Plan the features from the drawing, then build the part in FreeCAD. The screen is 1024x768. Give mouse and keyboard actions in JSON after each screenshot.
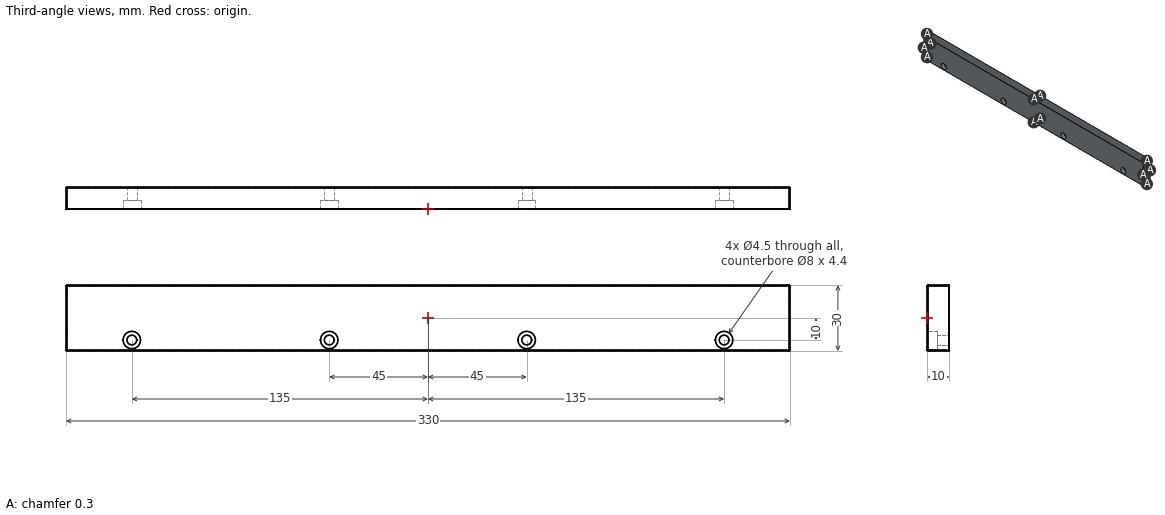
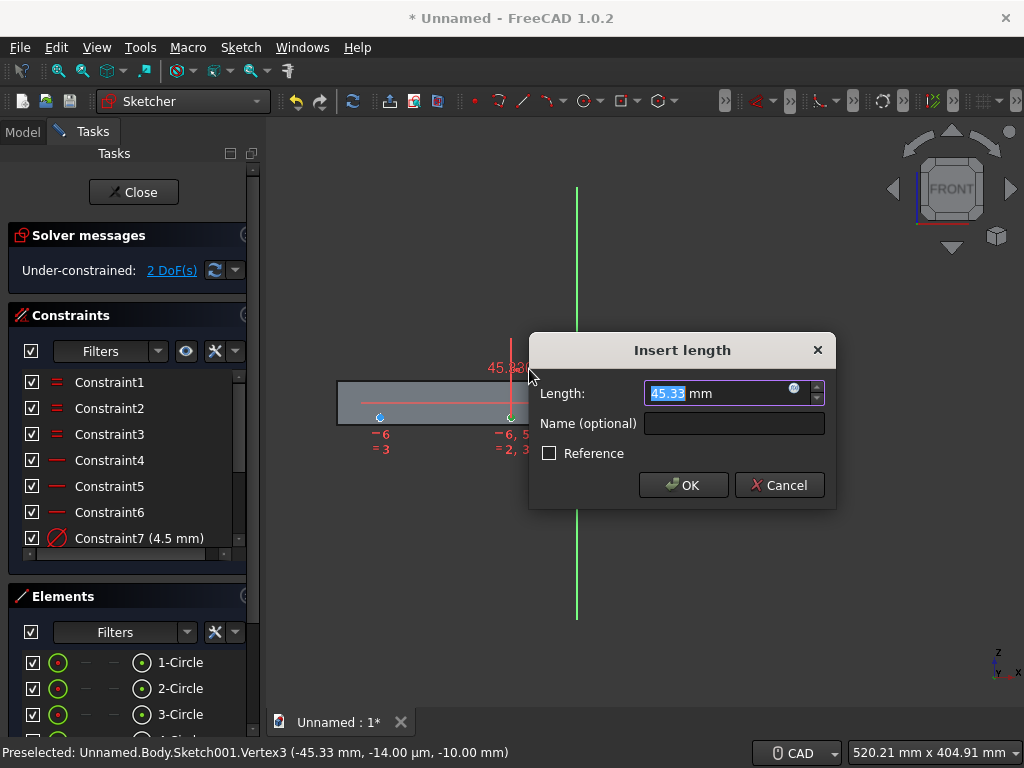
{"action": "type", "text": "45"}
{"action": "key", "text": "Return"}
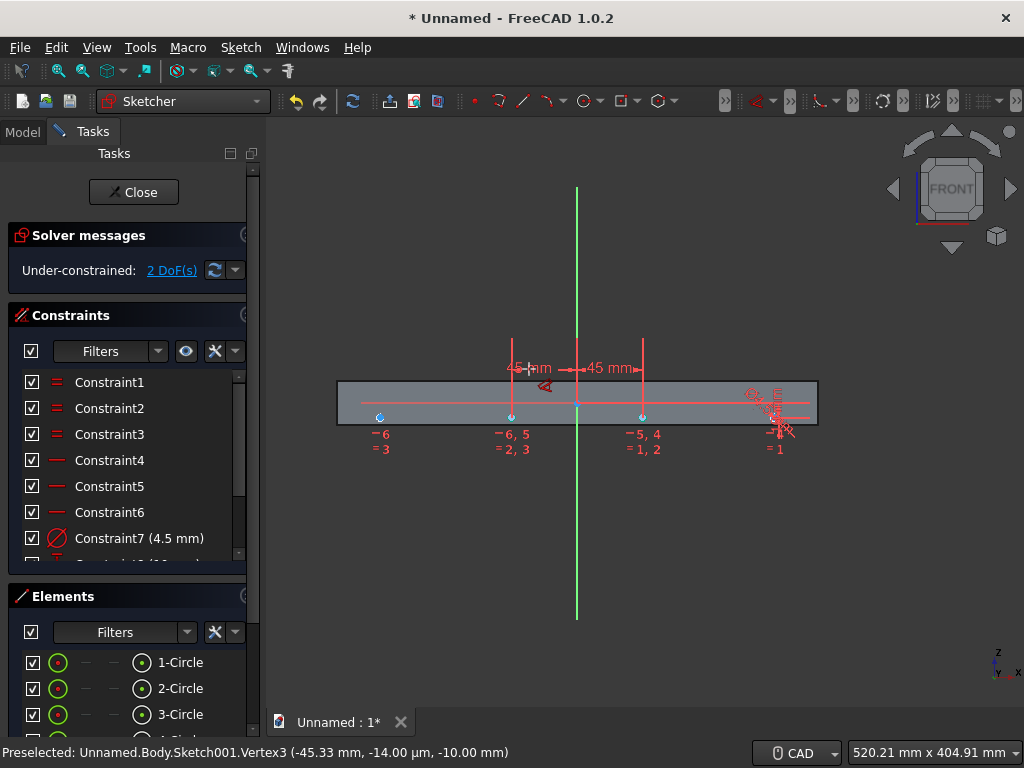
{"action": "left_click", "coordinate": [774, 418]}
{"action": "left_click", "coordinate": [721, 369]}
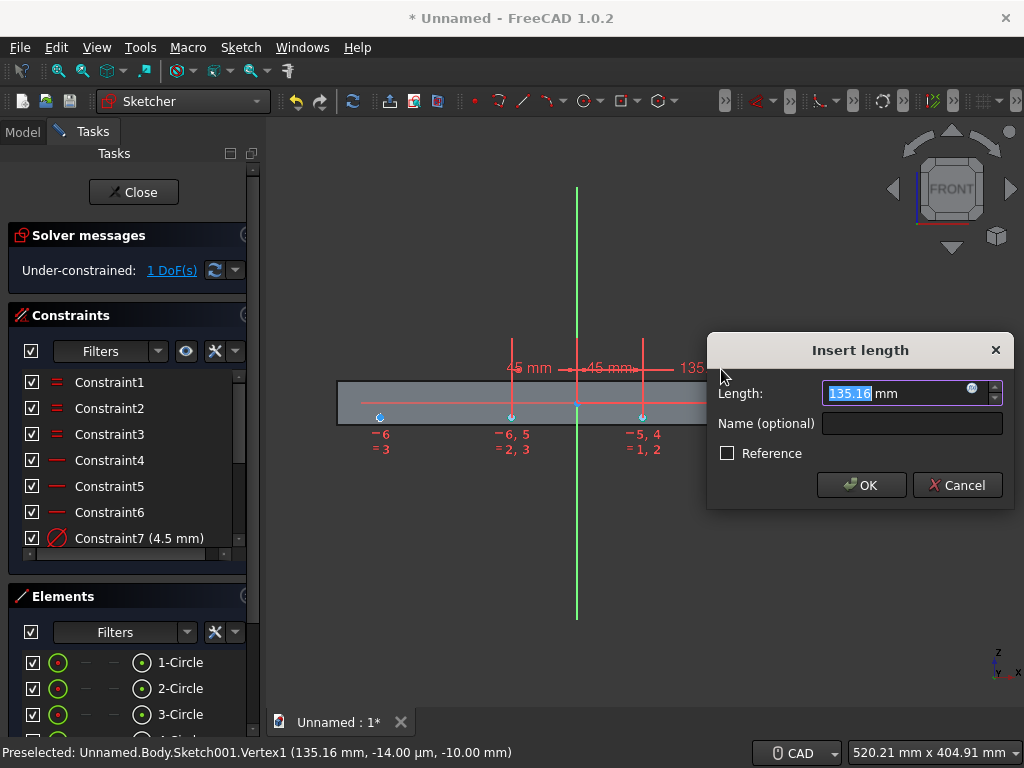
{"action": "type", "text": "135"}
{"action": "key", "text": "Return"}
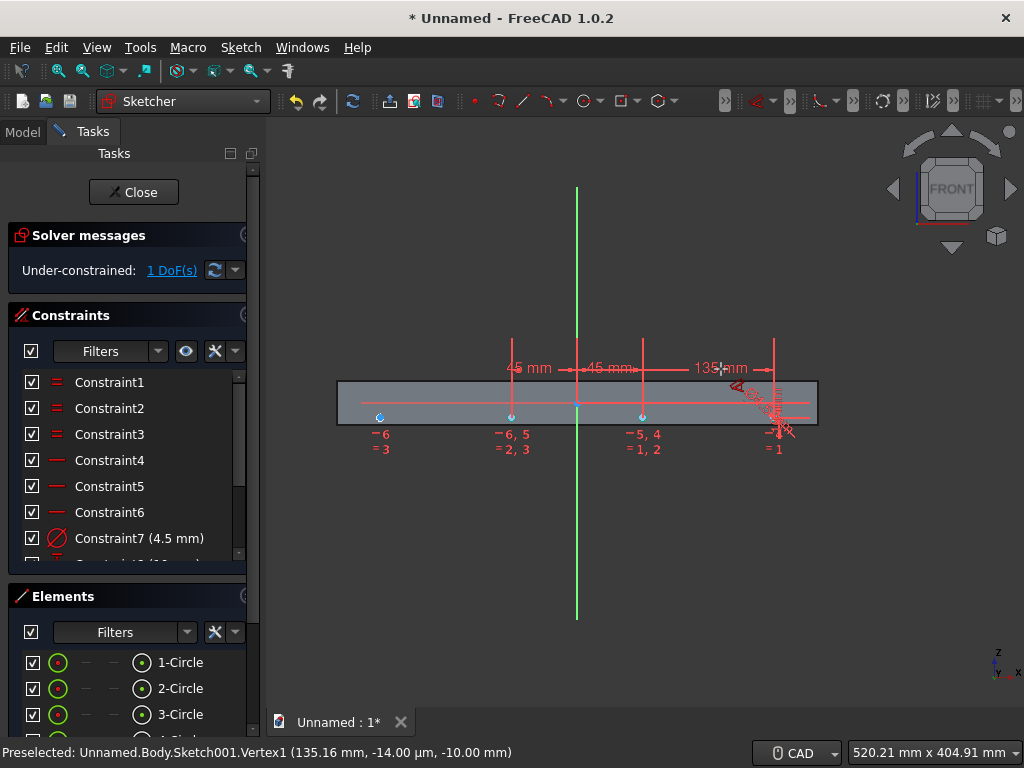
{"action": "left_click", "coordinate": [380, 418]}
{"action": "left_click", "coordinate": [433, 369]}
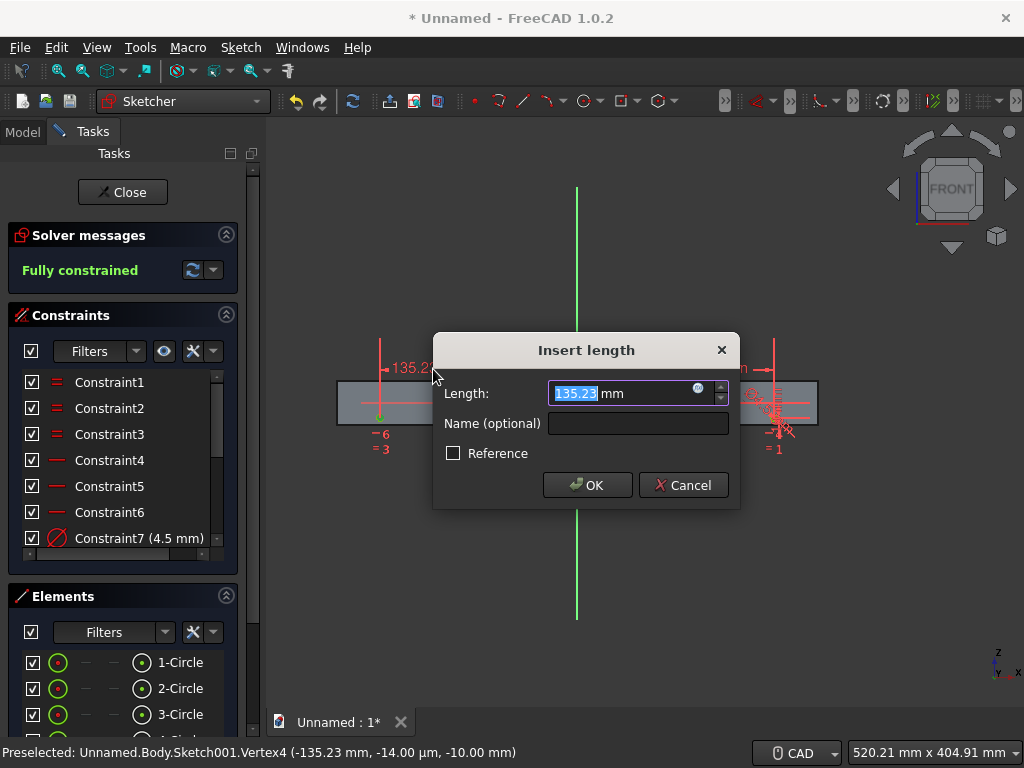
{"action": "type", "text": "135"}
{"action": "key", "text": "Return"}
{"action": "key", "text": "Escape"}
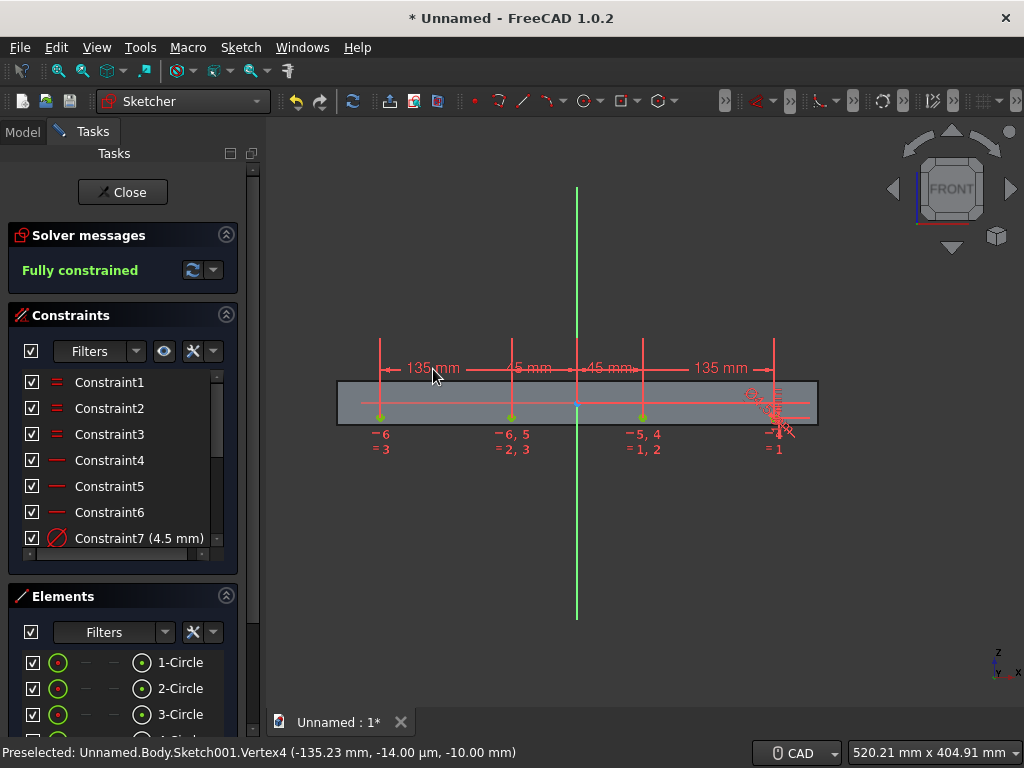
{"action": "left_click", "coordinate": [123, 192]}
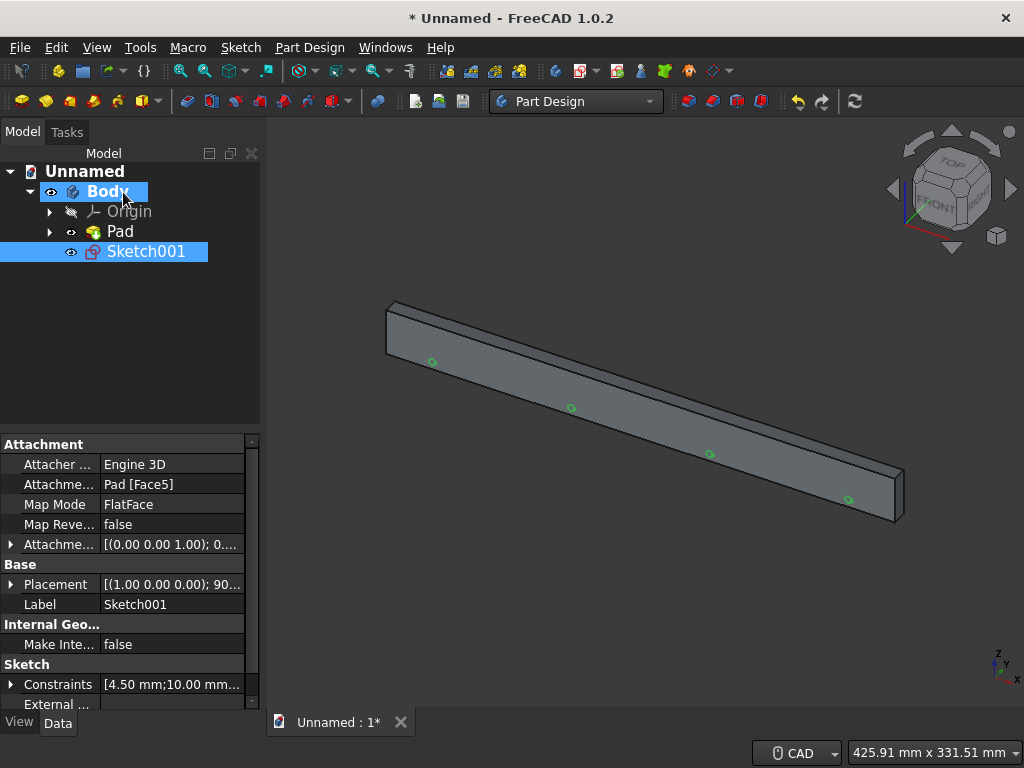
{"action": "left_click", "coordinate": [212, 102]}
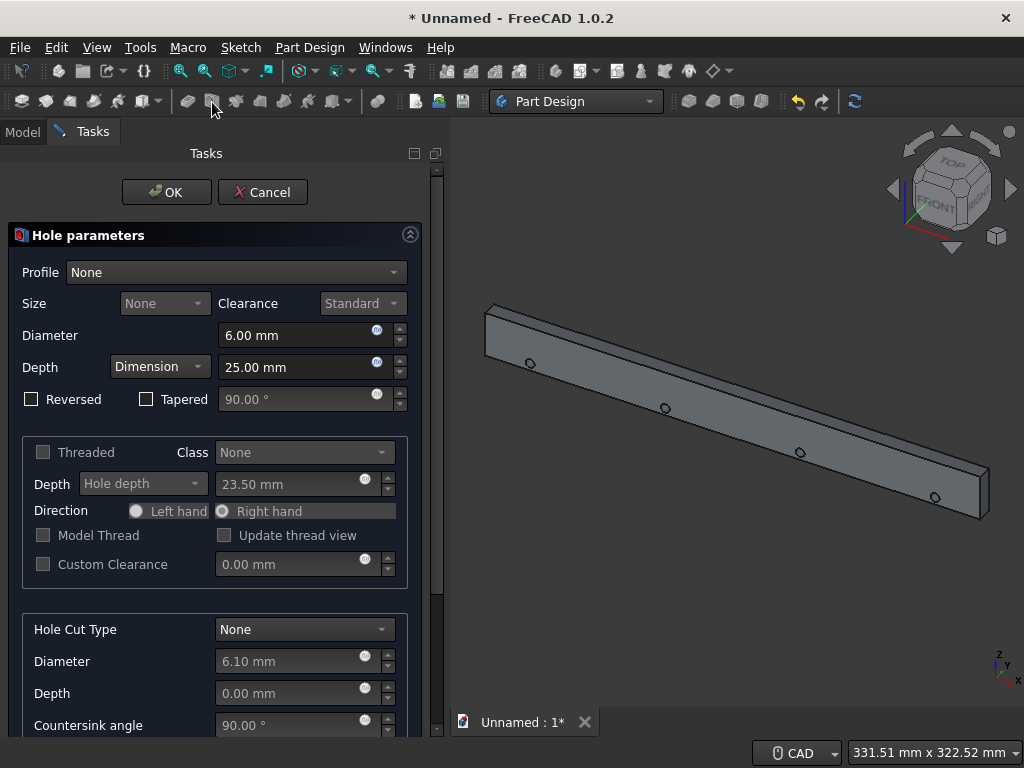
{"action": "triple_click", "coordinate": [305, 335]}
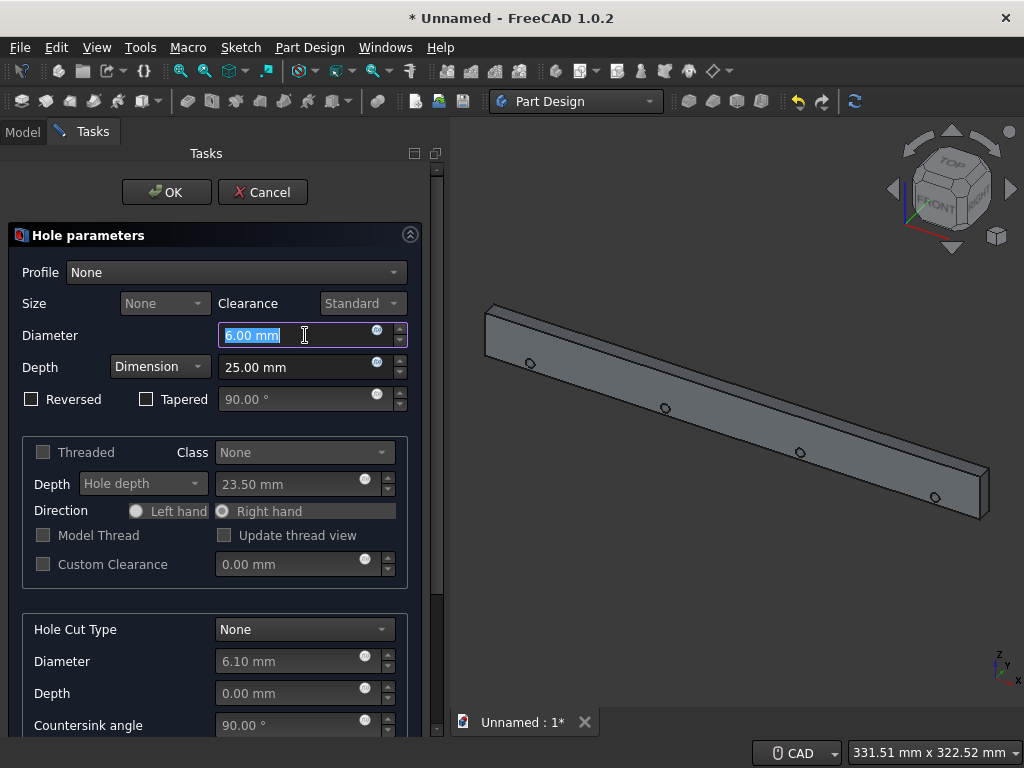
{"action": "type", "text": "4.5"}
{"action": "key", "text": "Tab"}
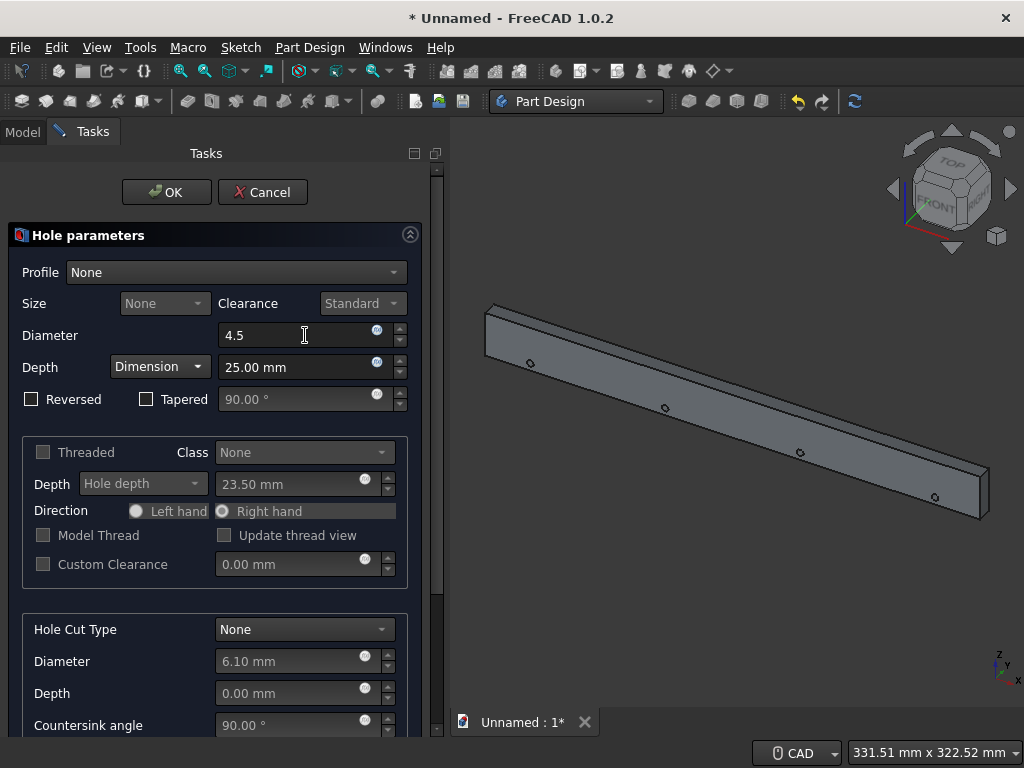
{"action": "left_click", "coordinate": [161, 366]}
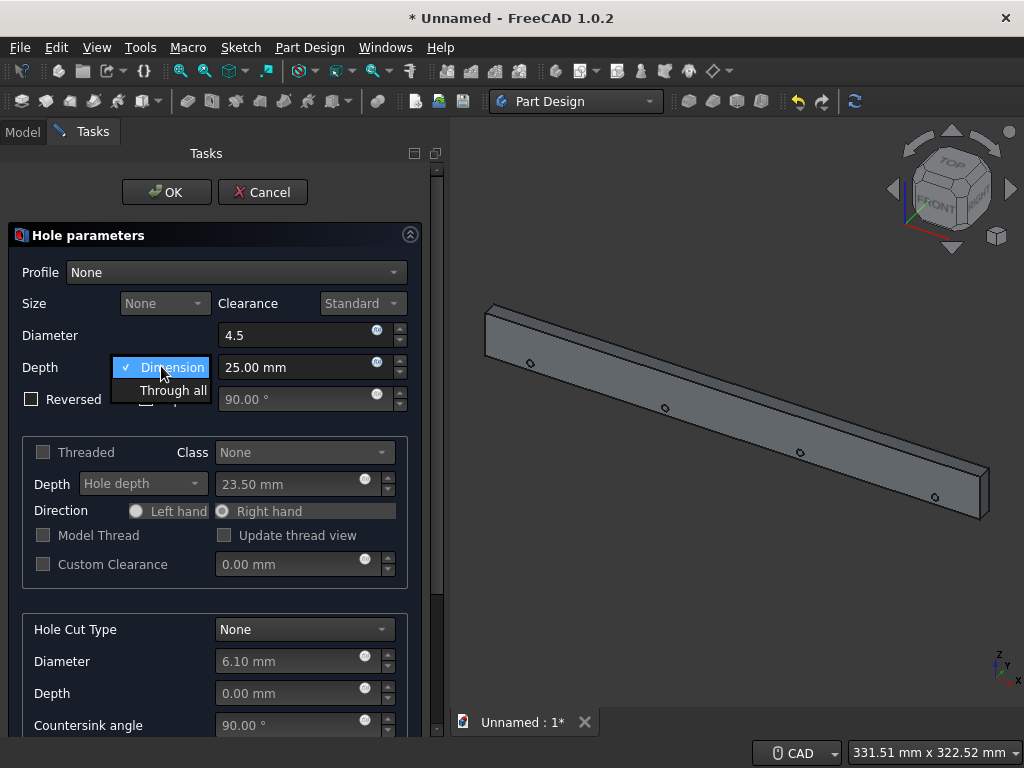
{"action": "left_click", "coordinate": [160, 390]}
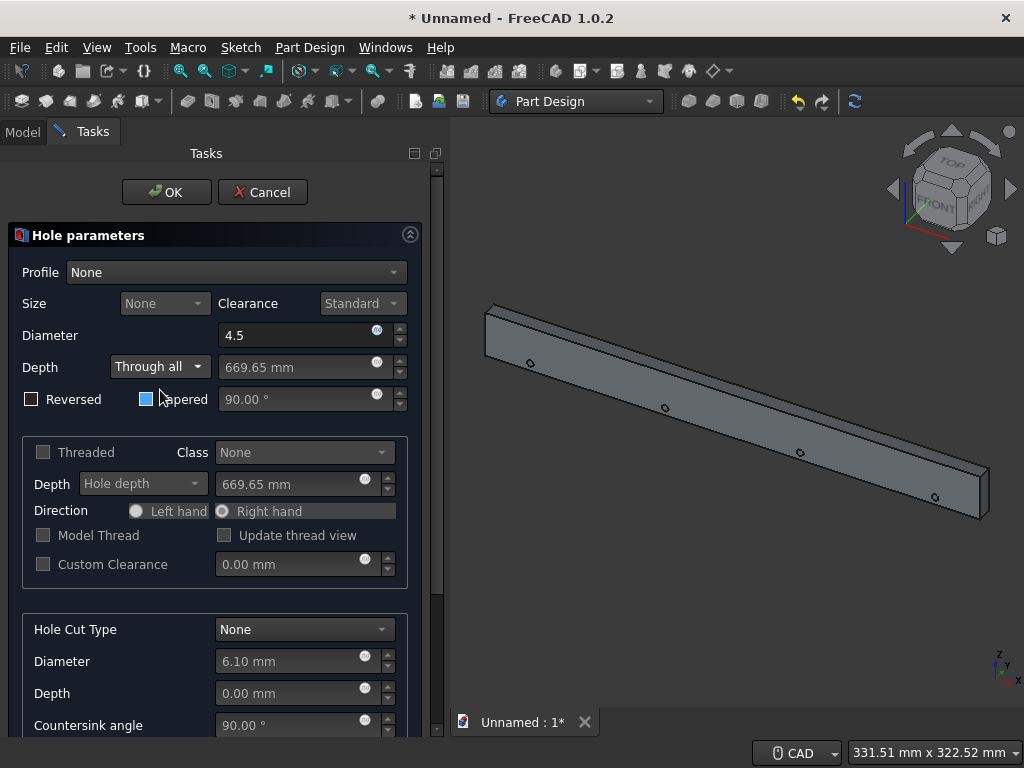
{"action": "left_click", "coordinate": [306, 630]}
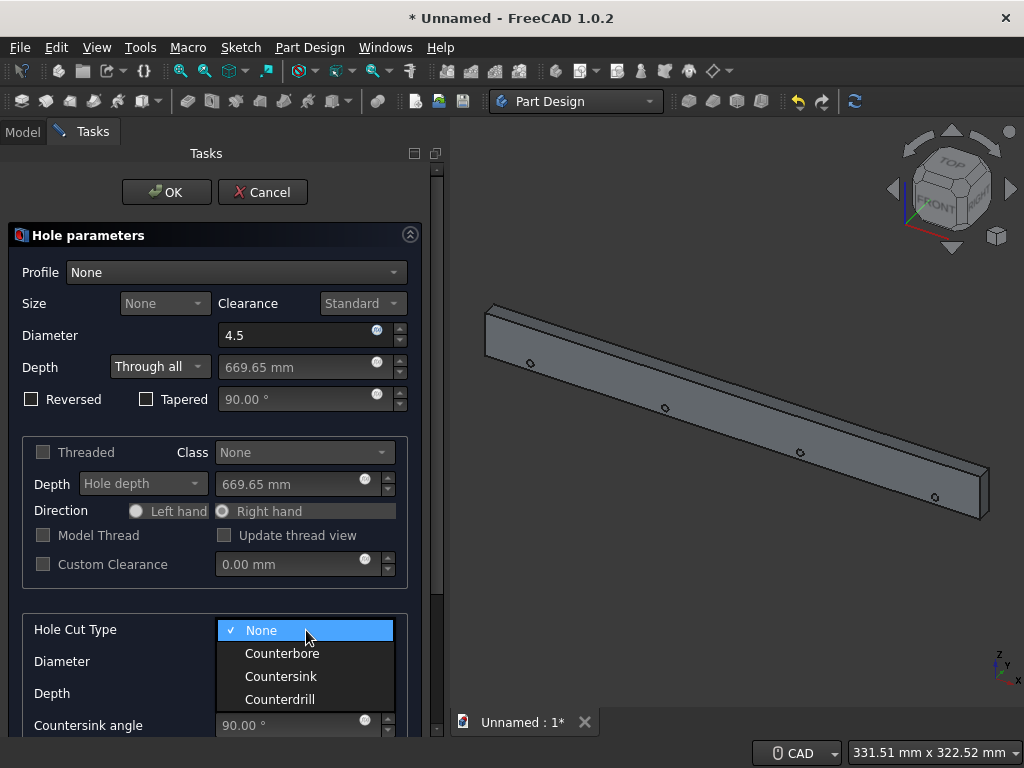
{"action": "left_click", "coordinate": [304, 654]}